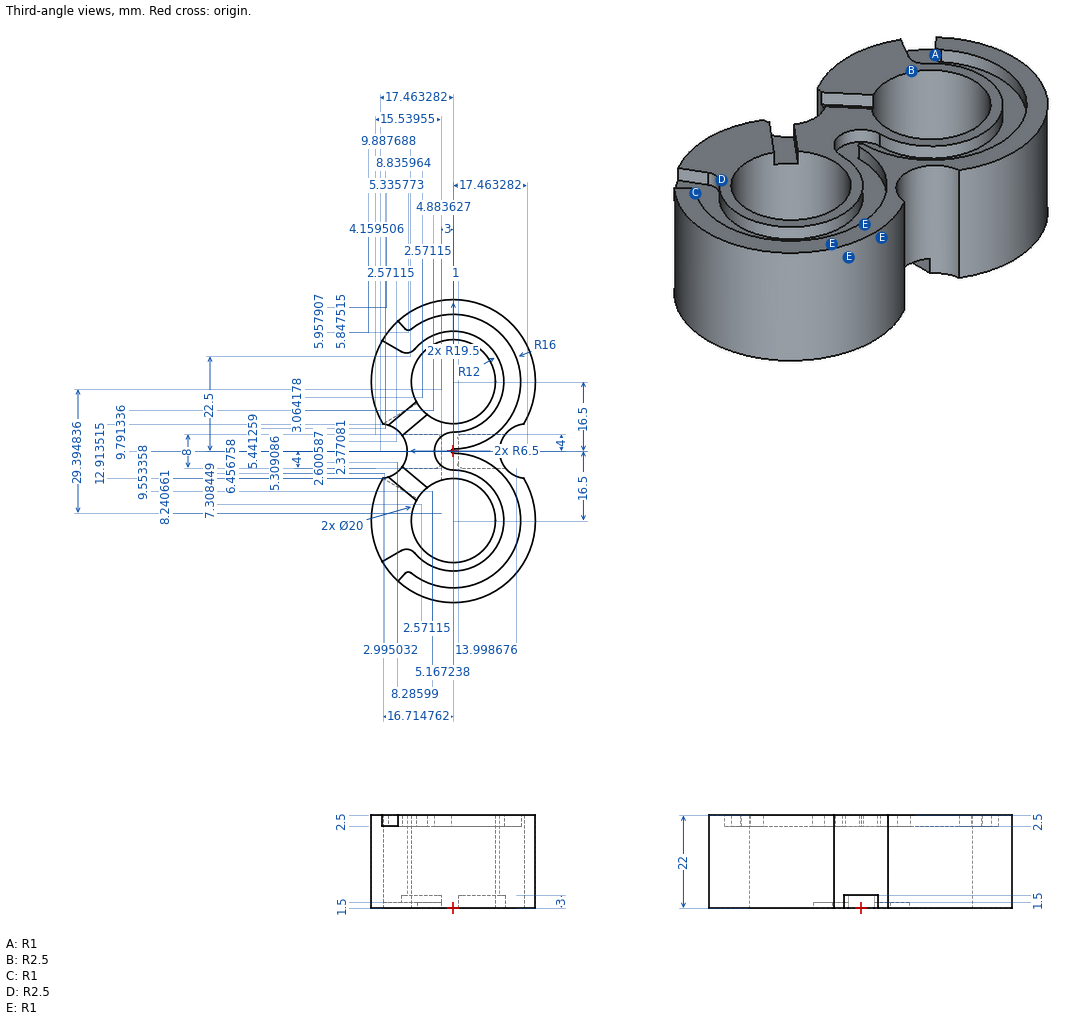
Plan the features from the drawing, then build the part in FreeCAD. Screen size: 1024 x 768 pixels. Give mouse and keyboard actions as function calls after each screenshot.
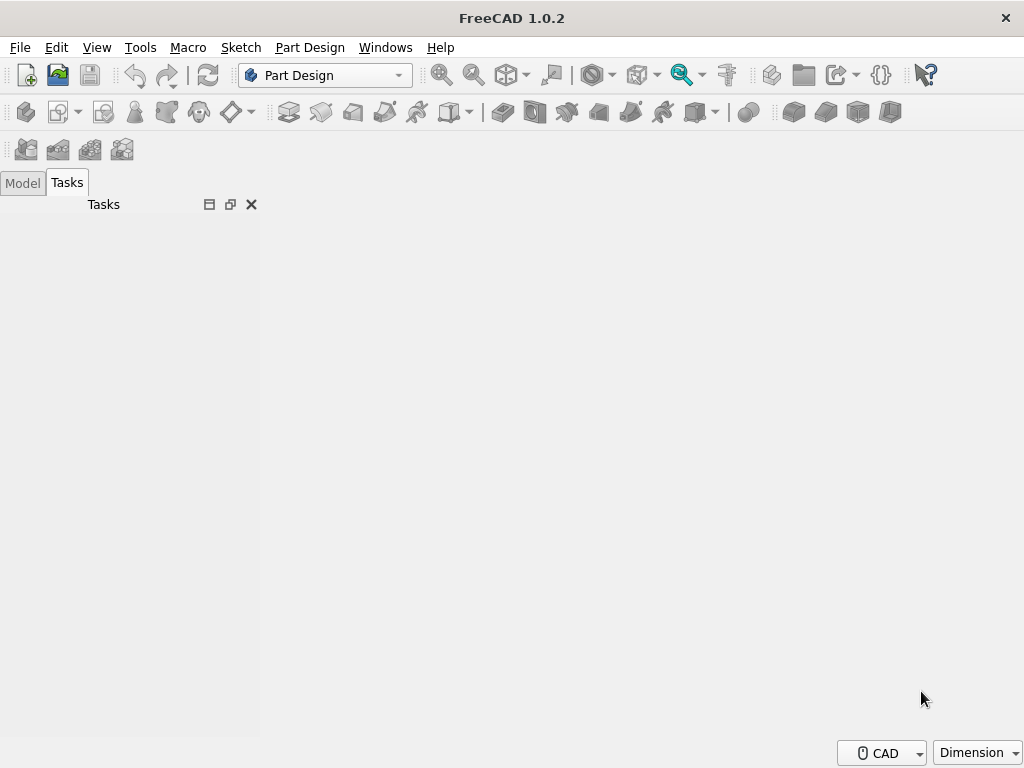
key(ctrl+n)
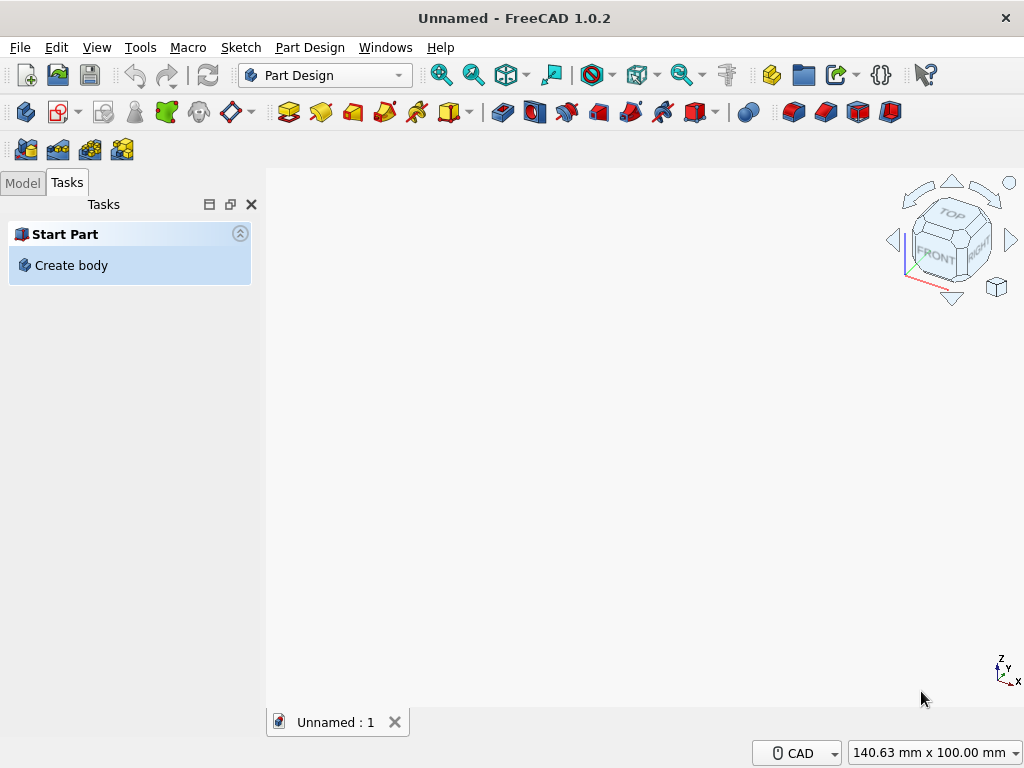
click(58, 112)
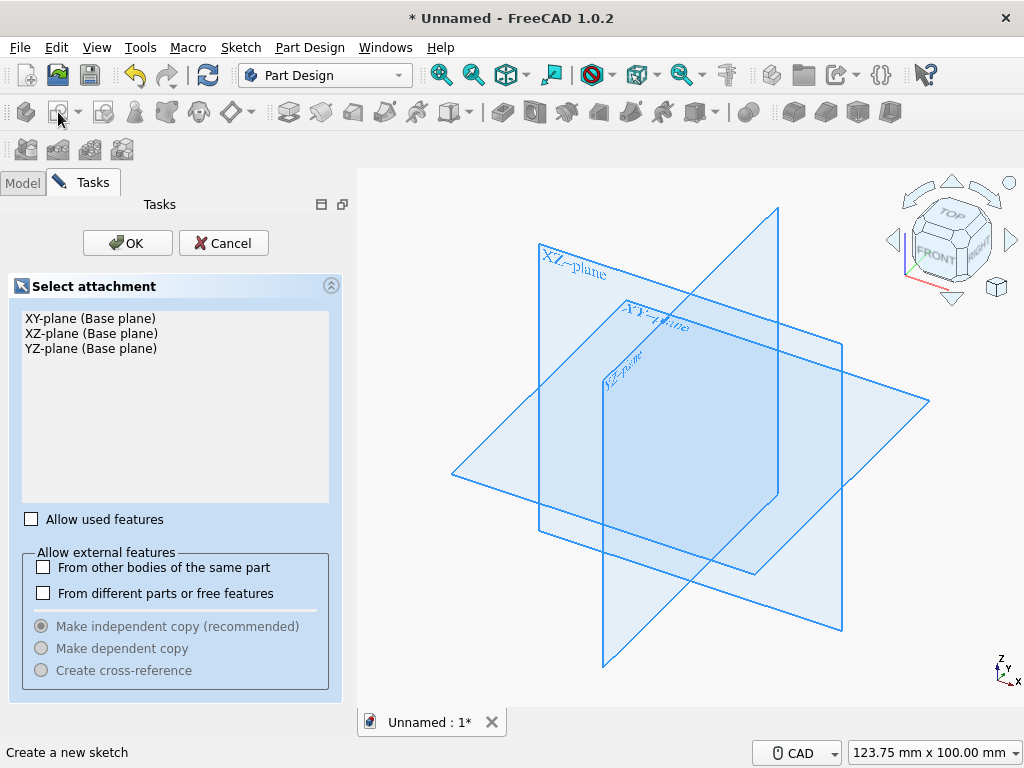
click(82, 318)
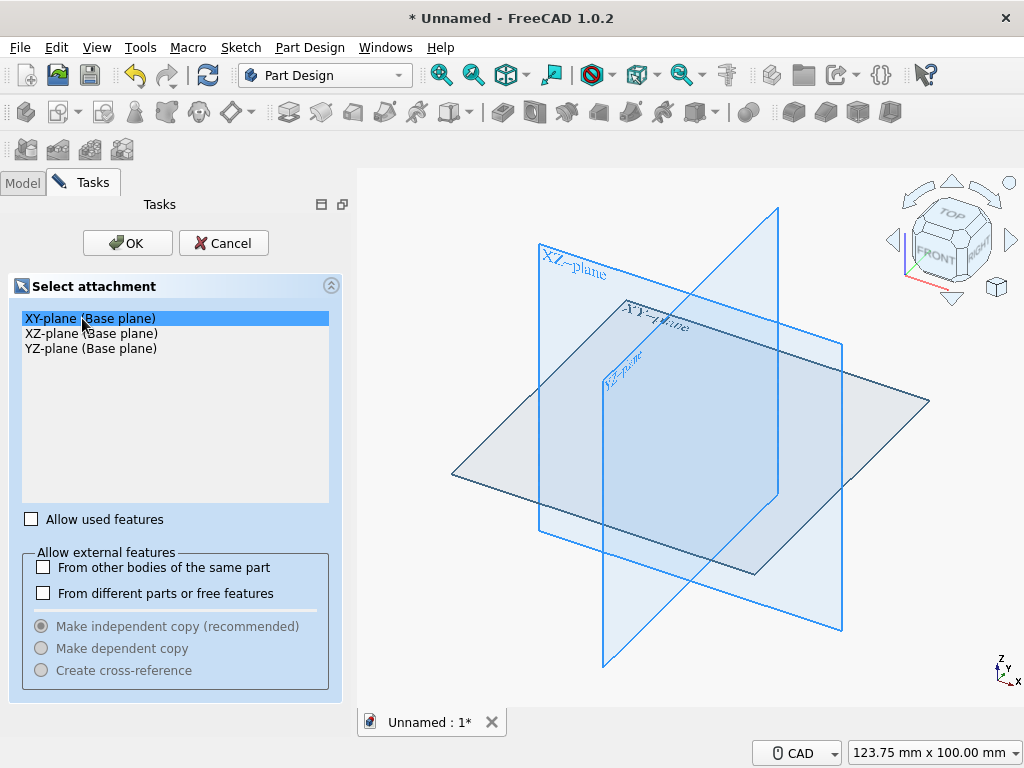
click(128, 243)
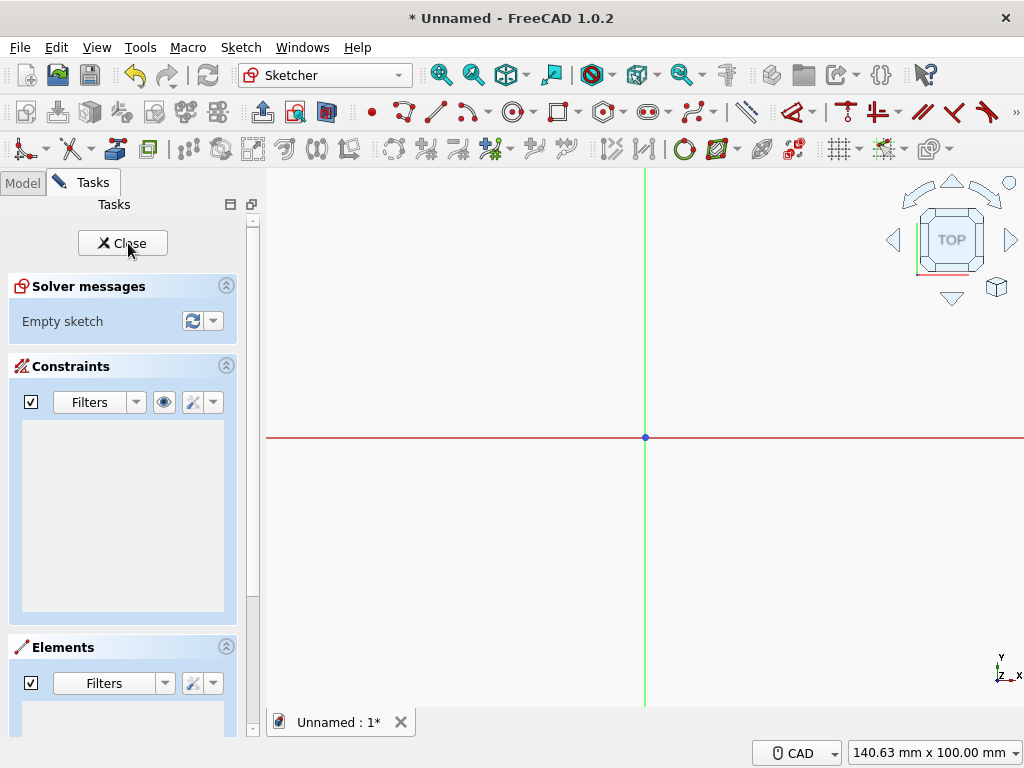
key(g)
key(3)
key(a)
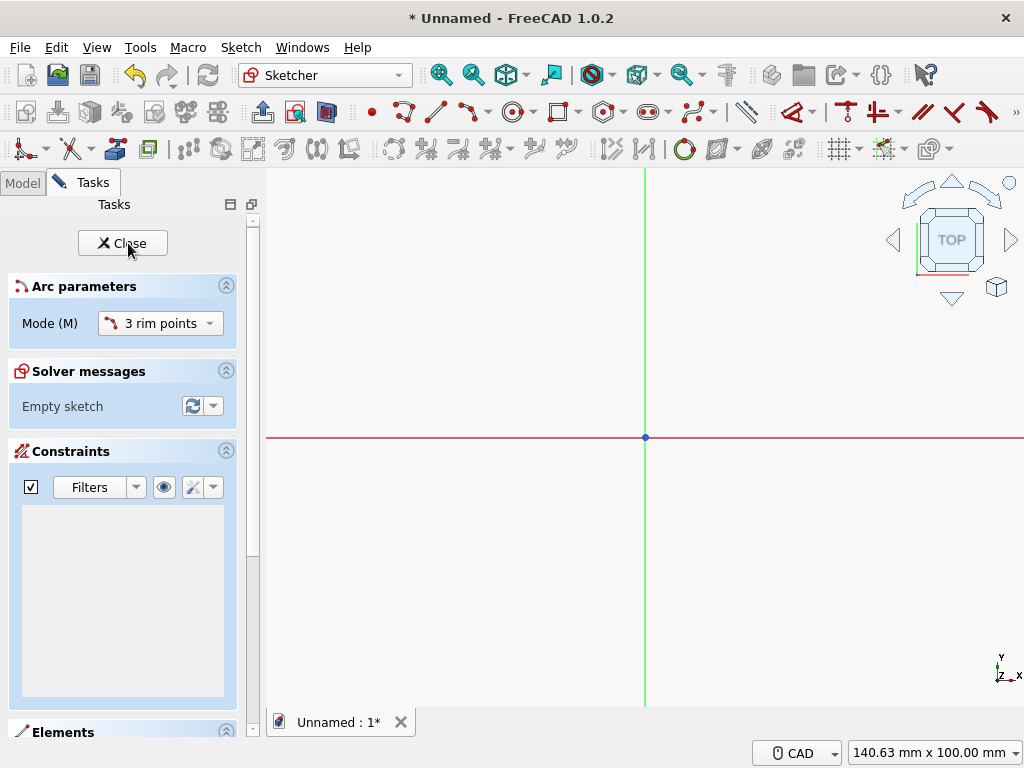
click(735, 403)
click(555, 403)
click(688, 253)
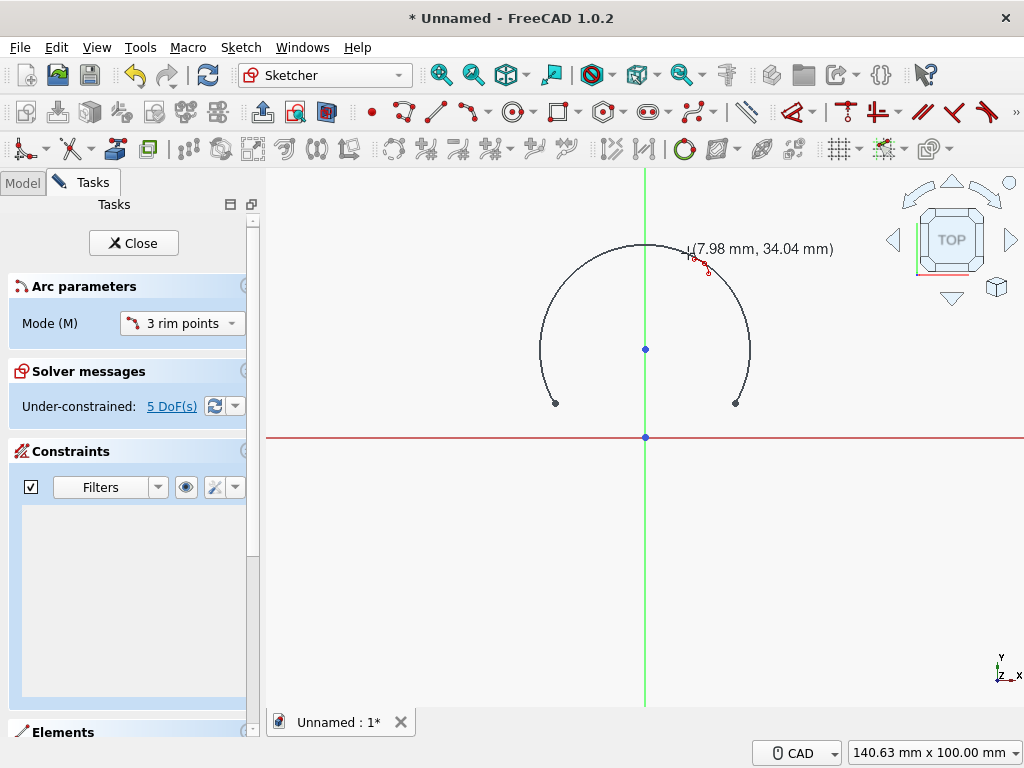
click(555, 404)
click(555, 472)
click(580, 457)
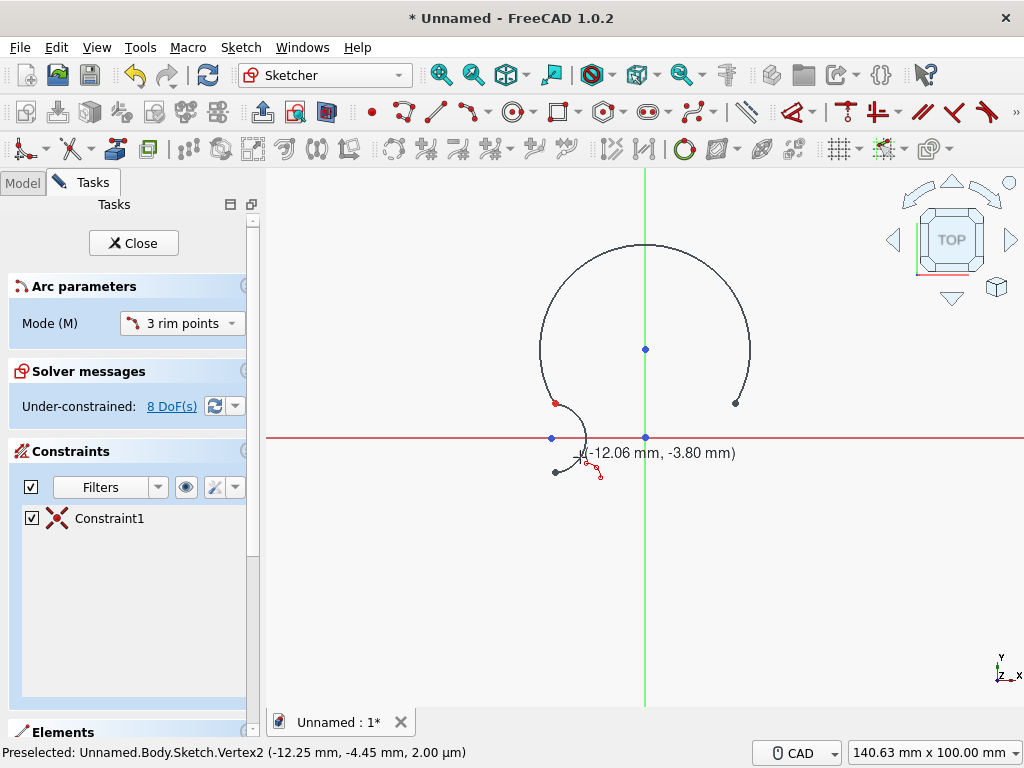
click(555, 473)
click(735, 472)
click(602, 622)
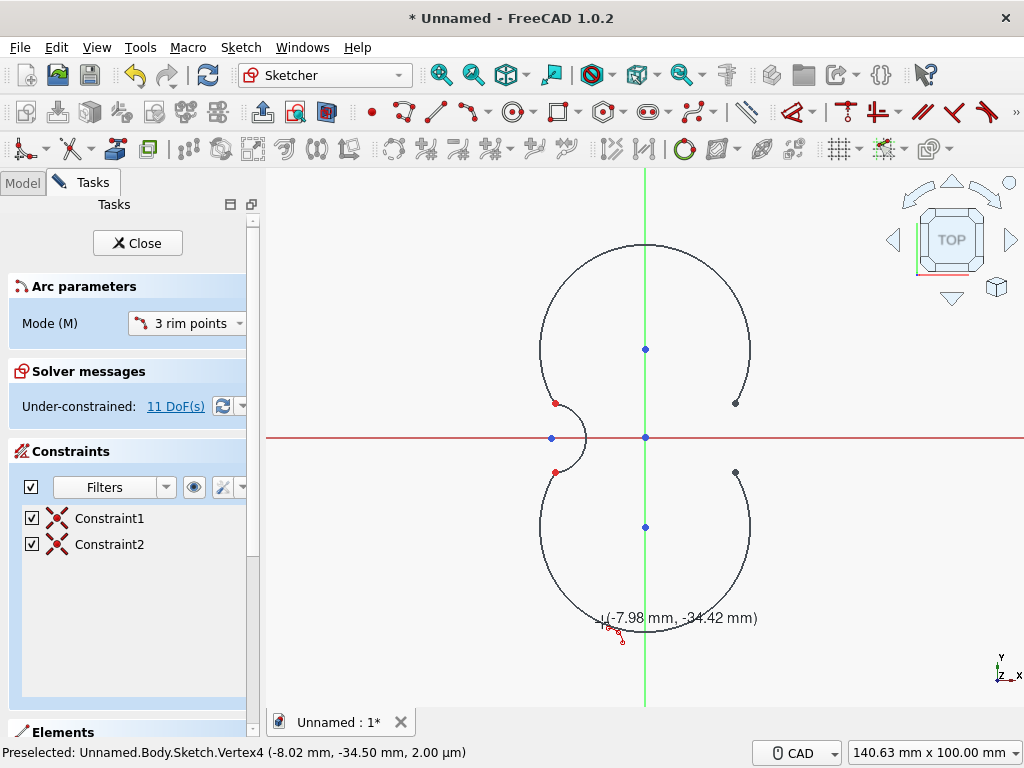
click(735, 473)
click(735, 404)
click(710, 418)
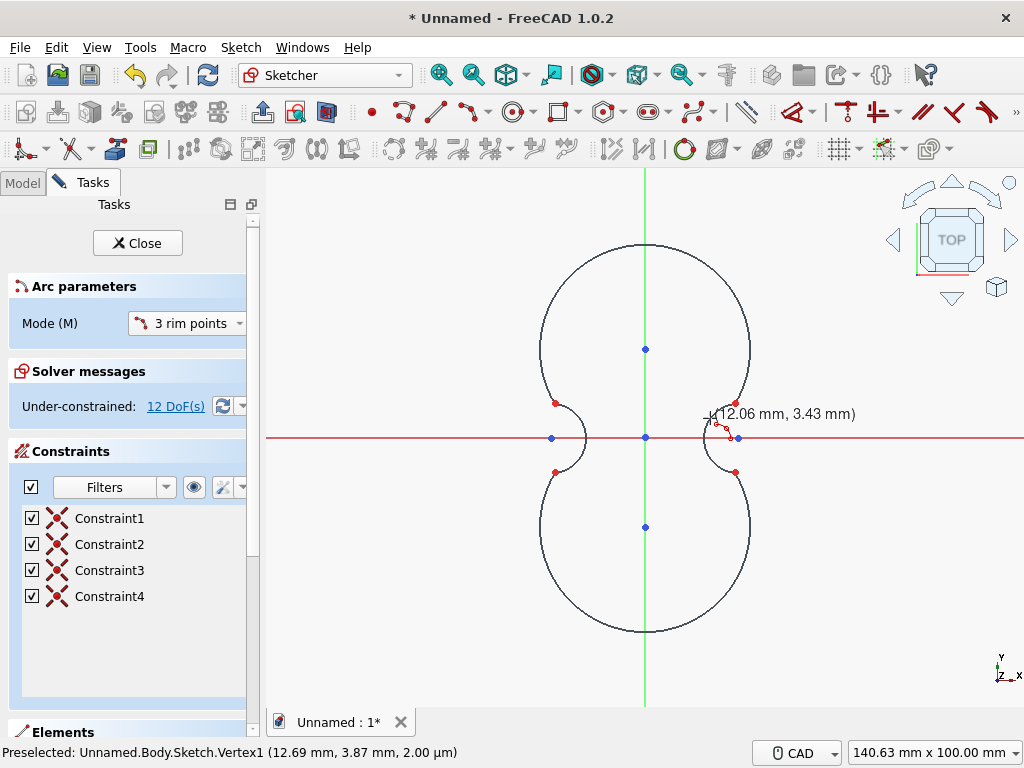
click(514, 112)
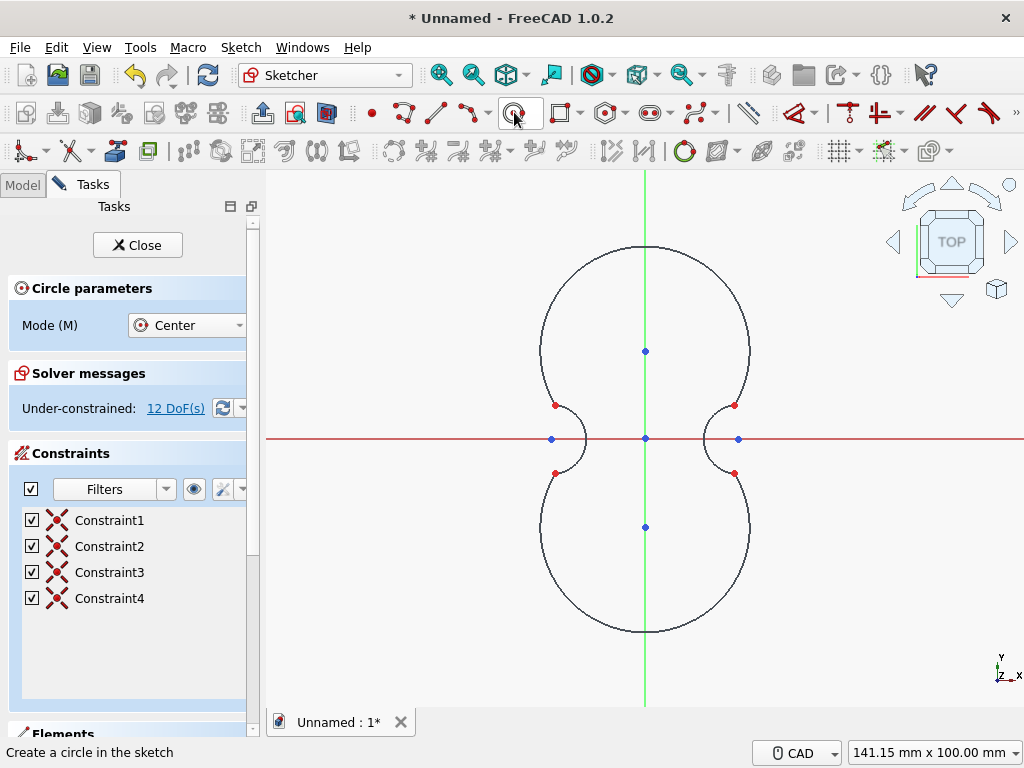
click(645, 527)
move(683, 489)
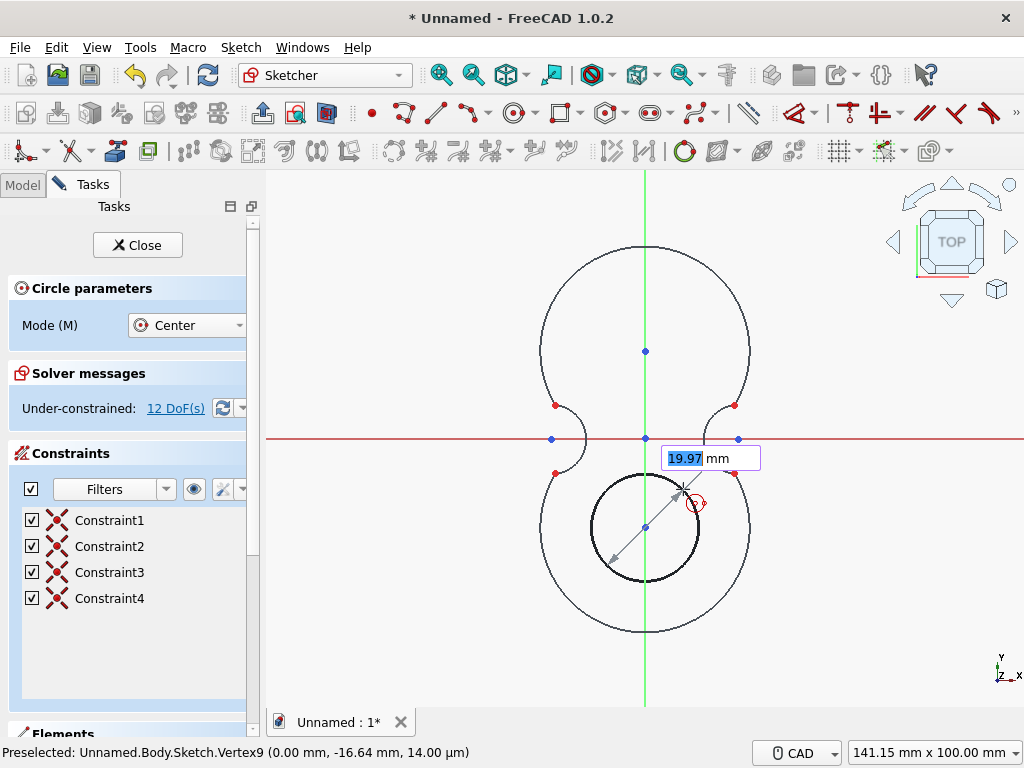
text(20)
key(Return)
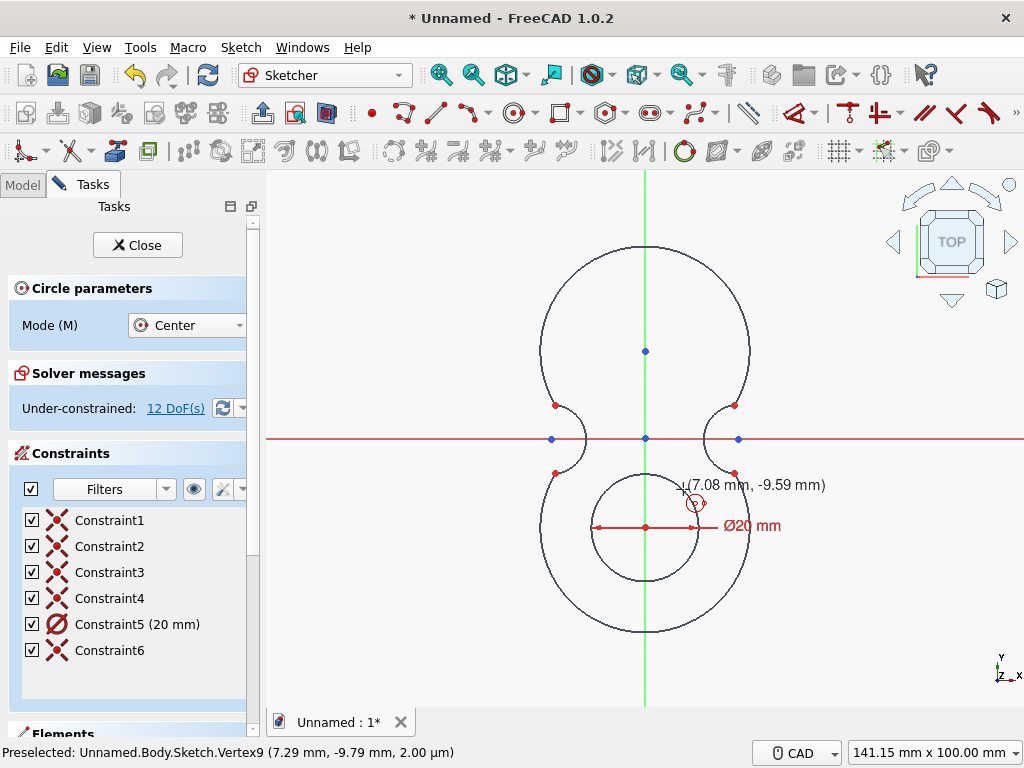
click(645, 350)
move(683, 312)